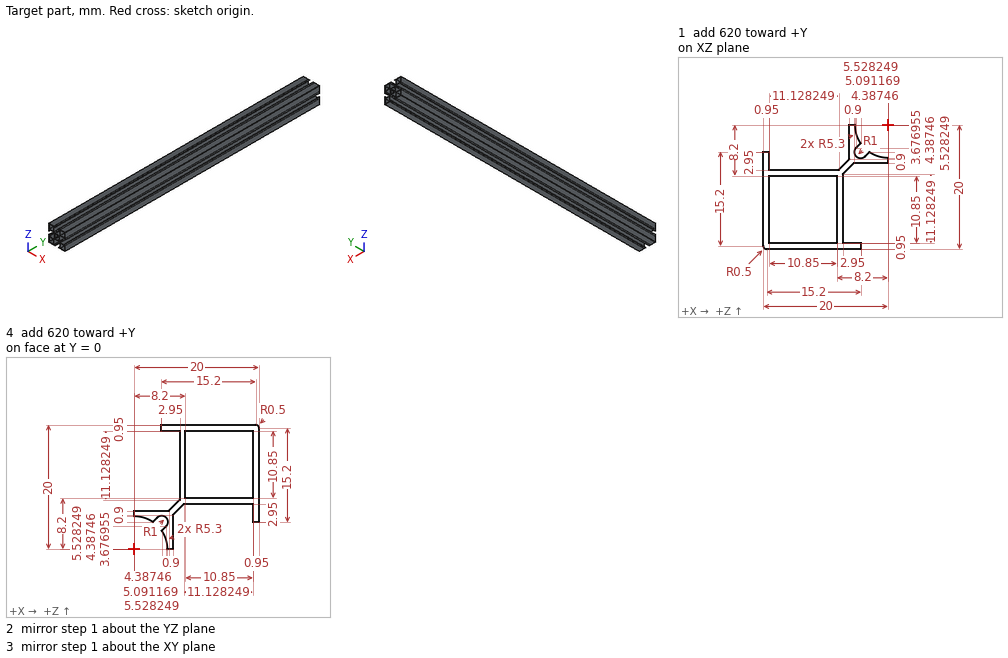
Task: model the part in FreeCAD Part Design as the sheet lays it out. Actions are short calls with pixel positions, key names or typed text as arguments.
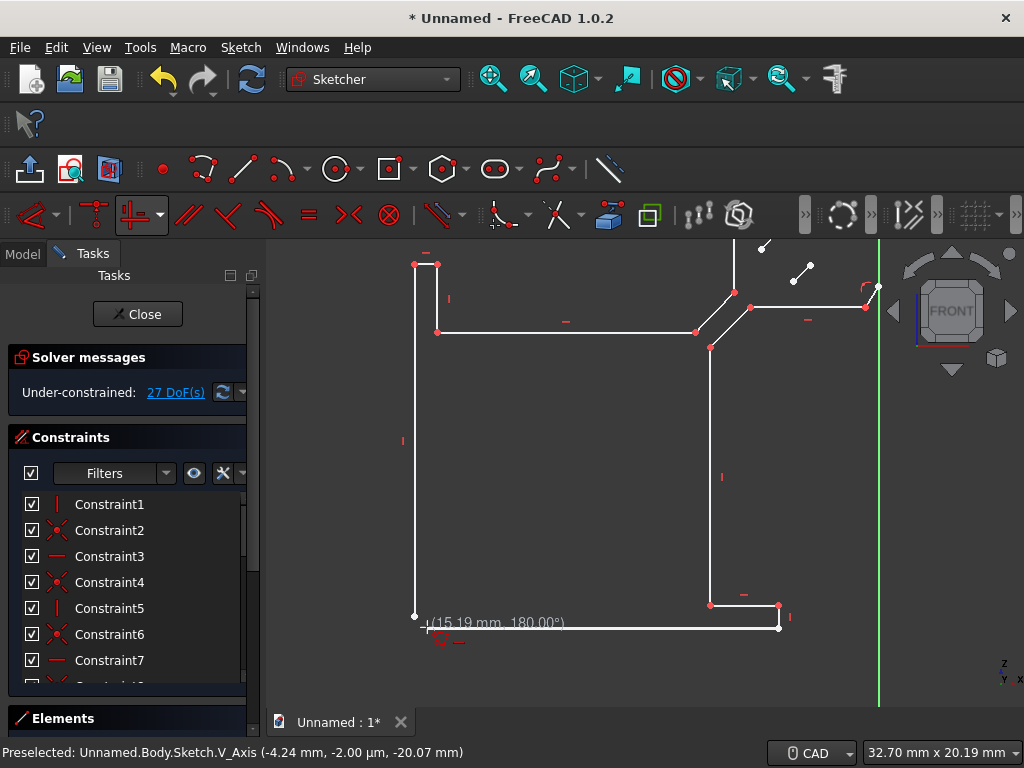
click(427, 627)
right_click(427, 627)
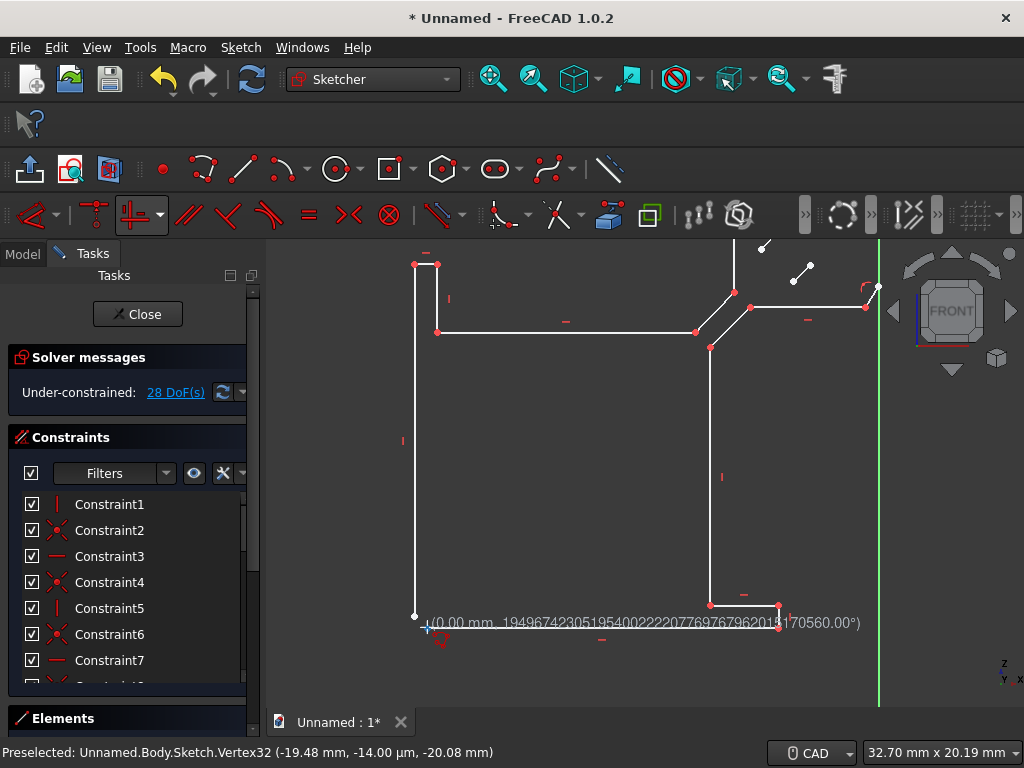
key(g)
key(3)
key(a)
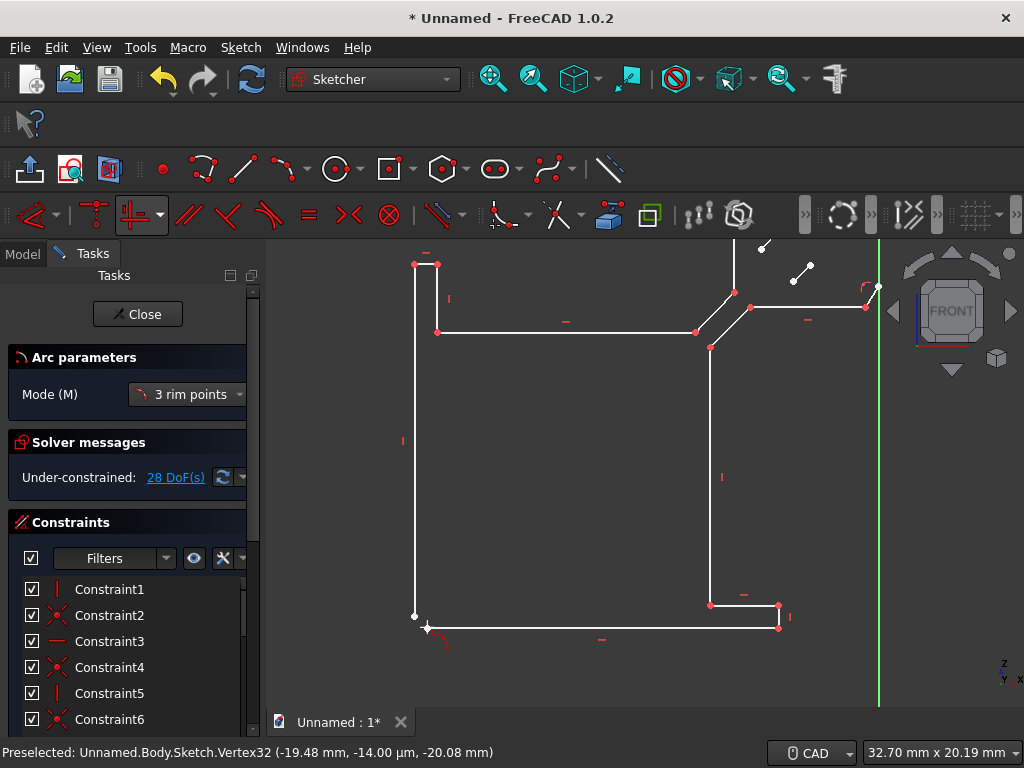
scroll(434, 633, down, 2)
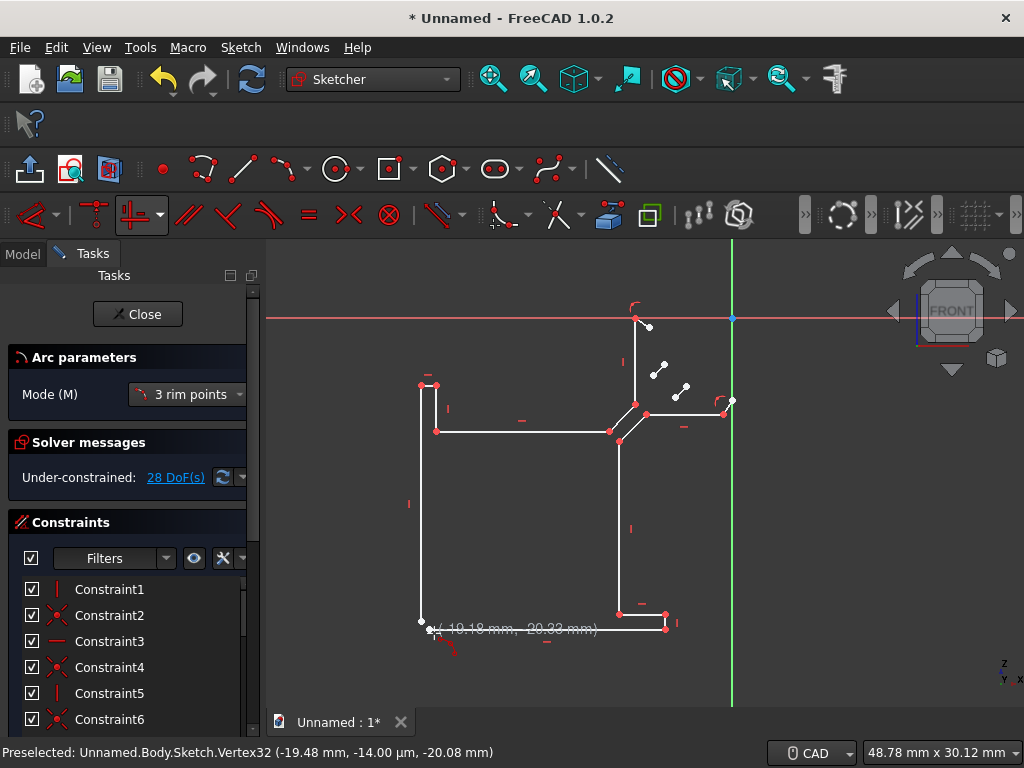
scroll(650, 318, up, 5)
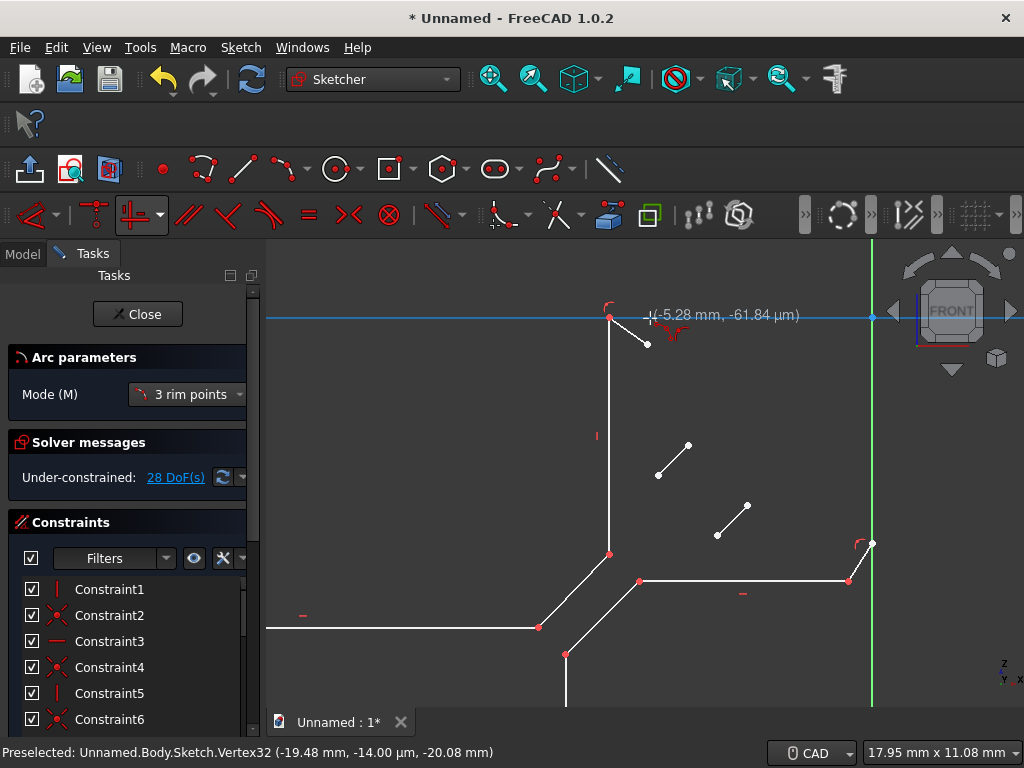
click(647, 345)
click(688, 445)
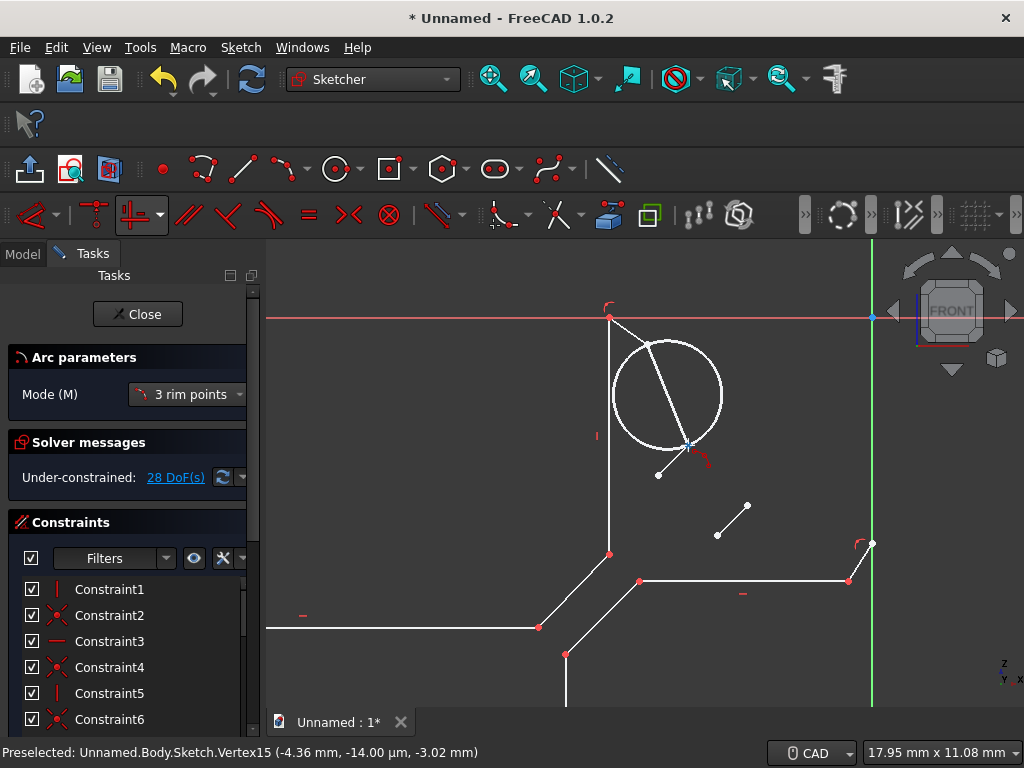
scroll(658, 383, up, 3)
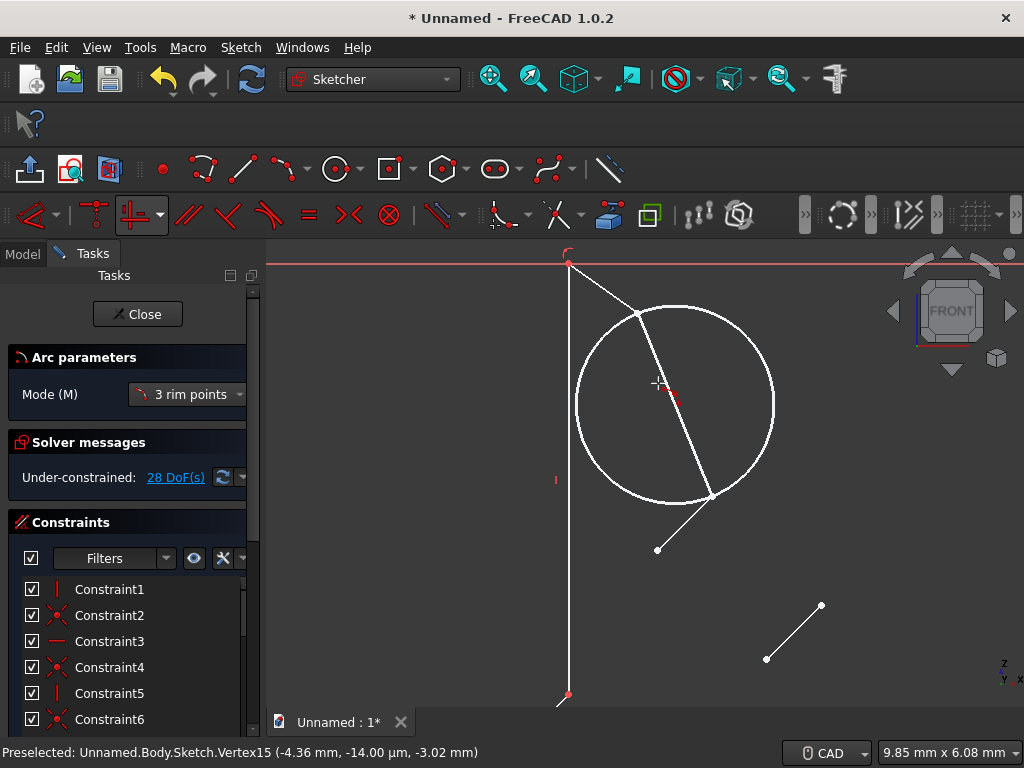
click(658, 384)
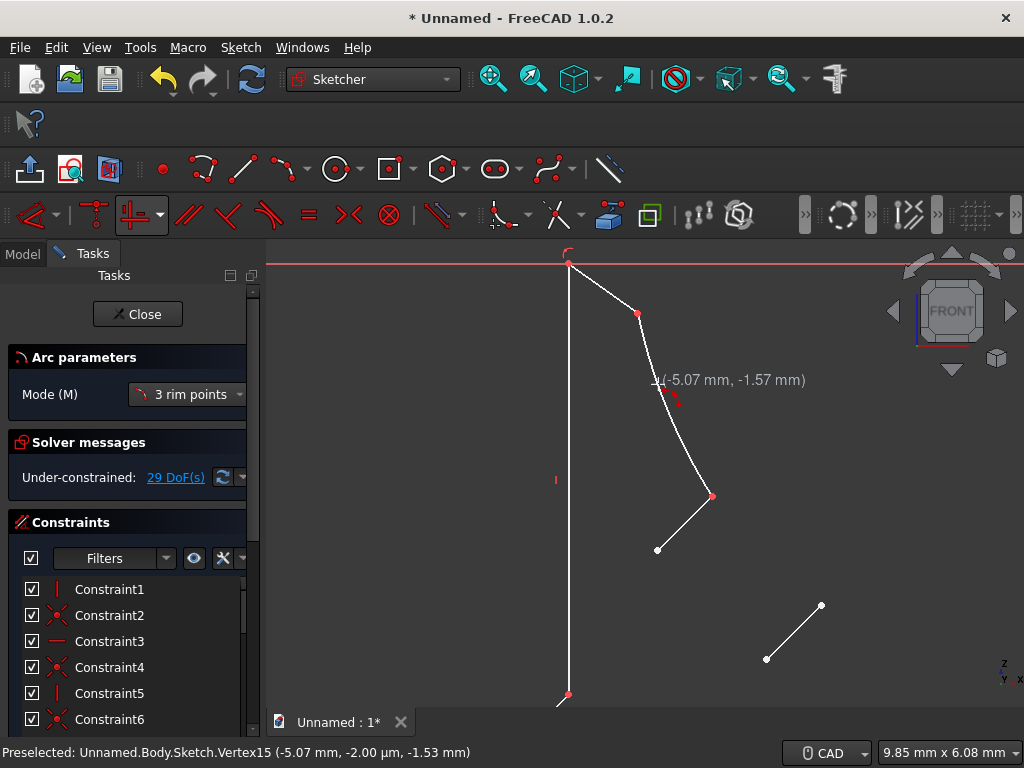
click(658, 551)
click(767, 660)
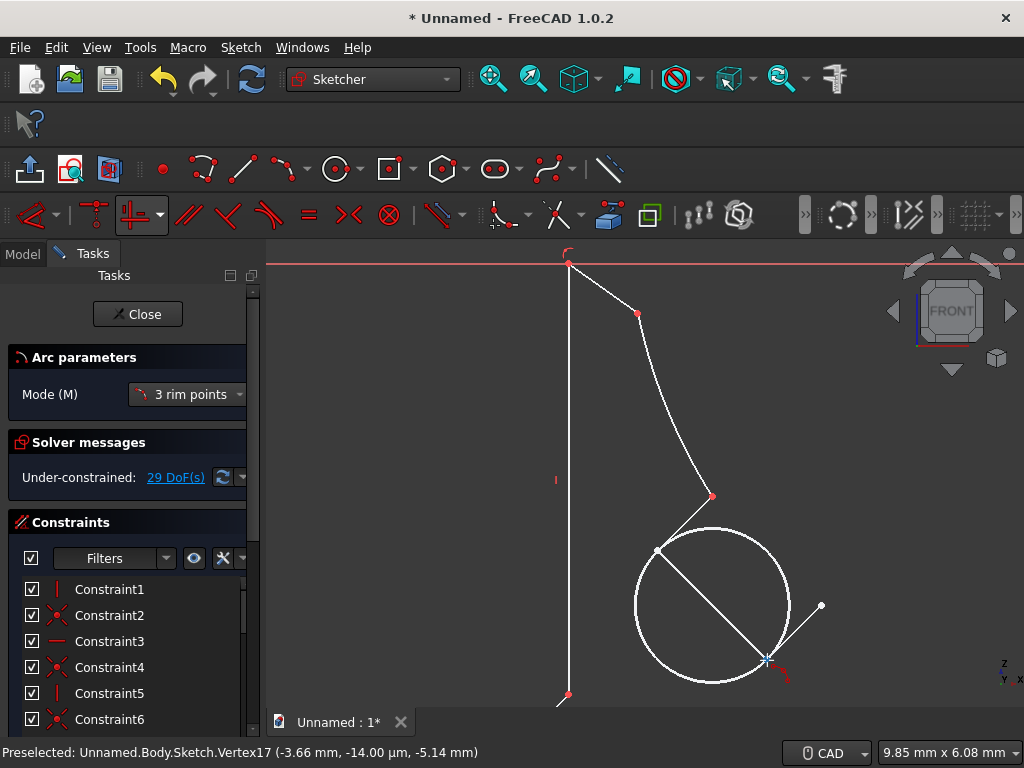
scroll(652, 331, down, 8)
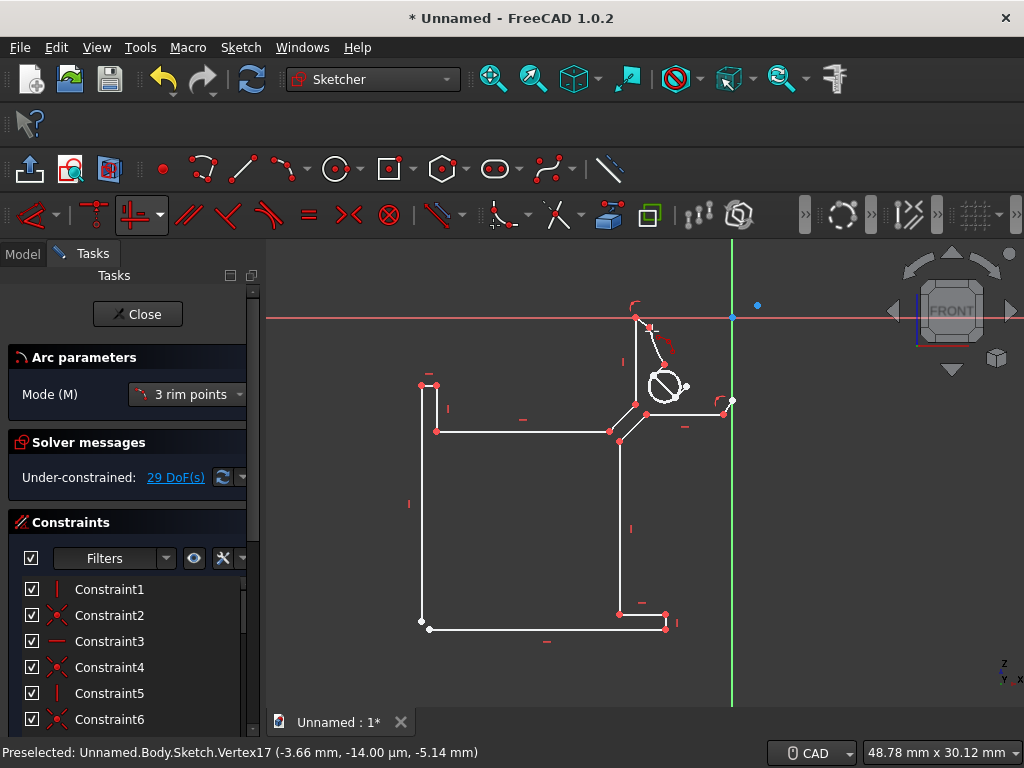
click(653, 397)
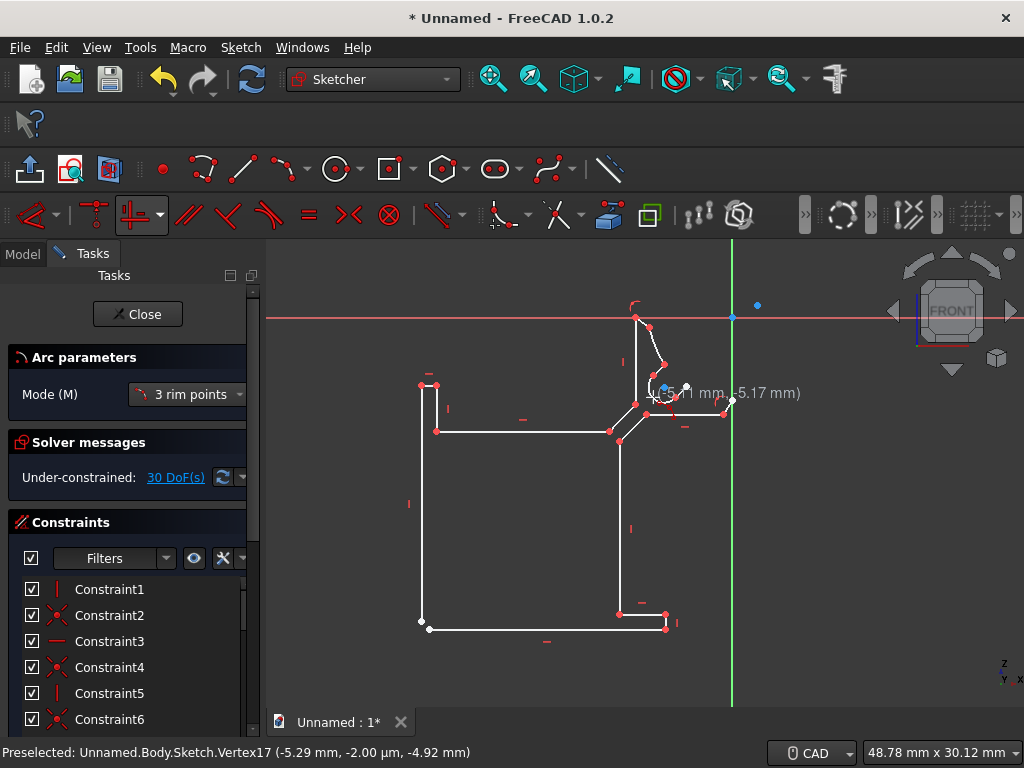
scroll(686, 386, up, 4)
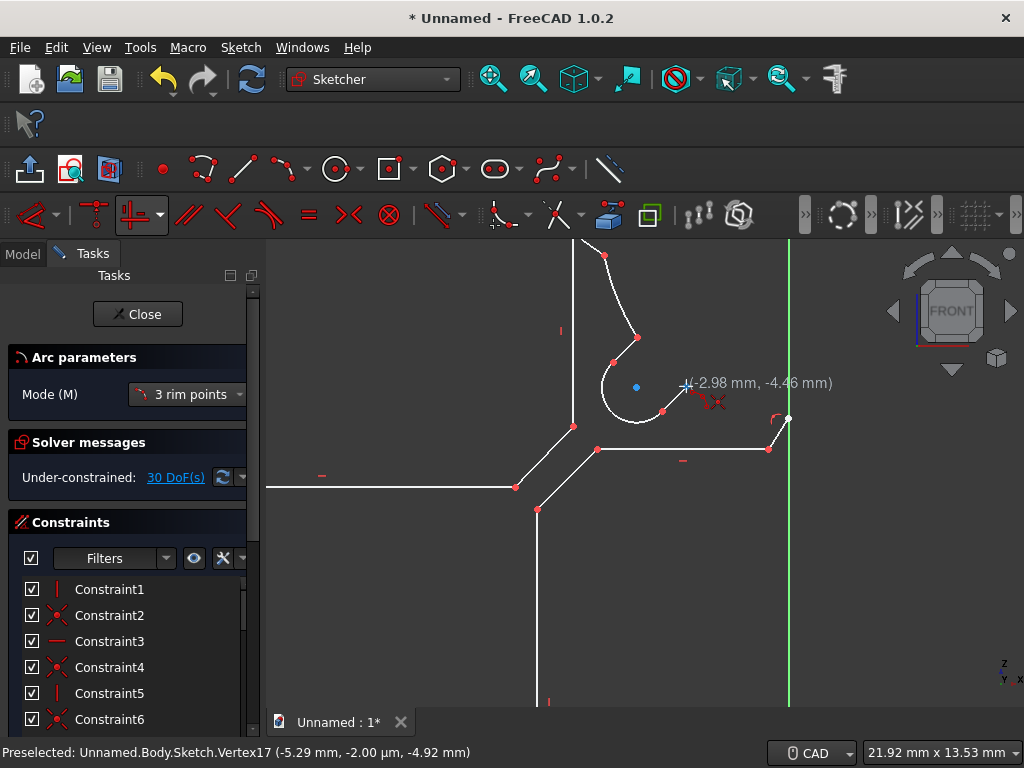
click(687, 387)
click(789, 418)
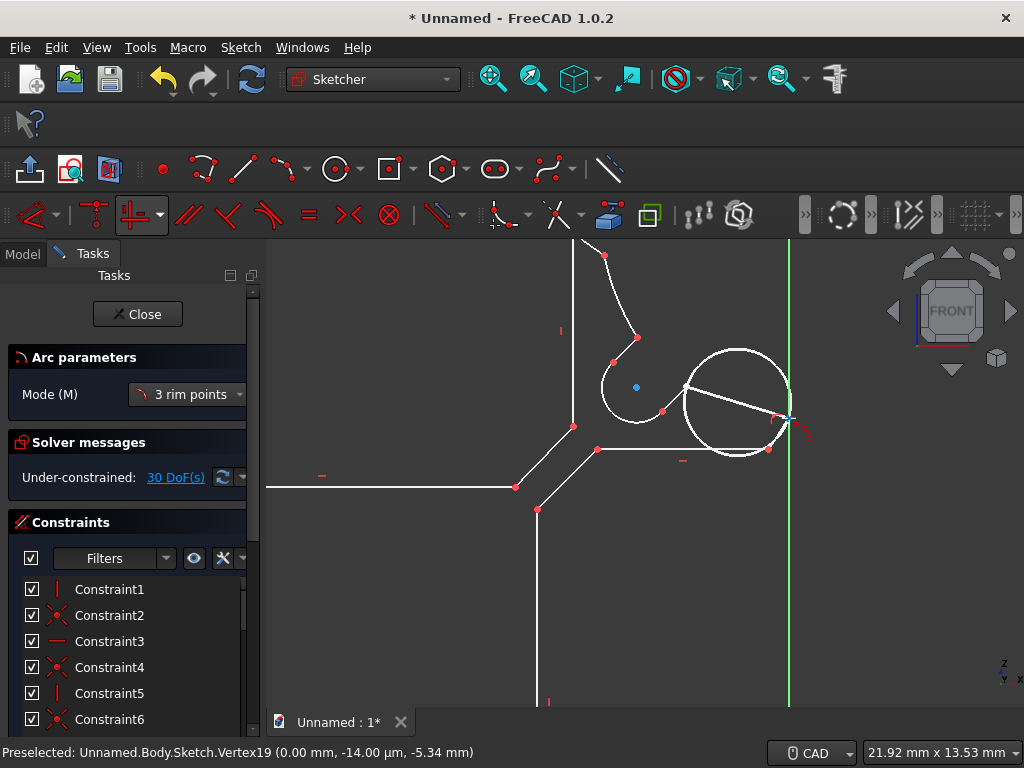
scroll(735, 409, up, 4)